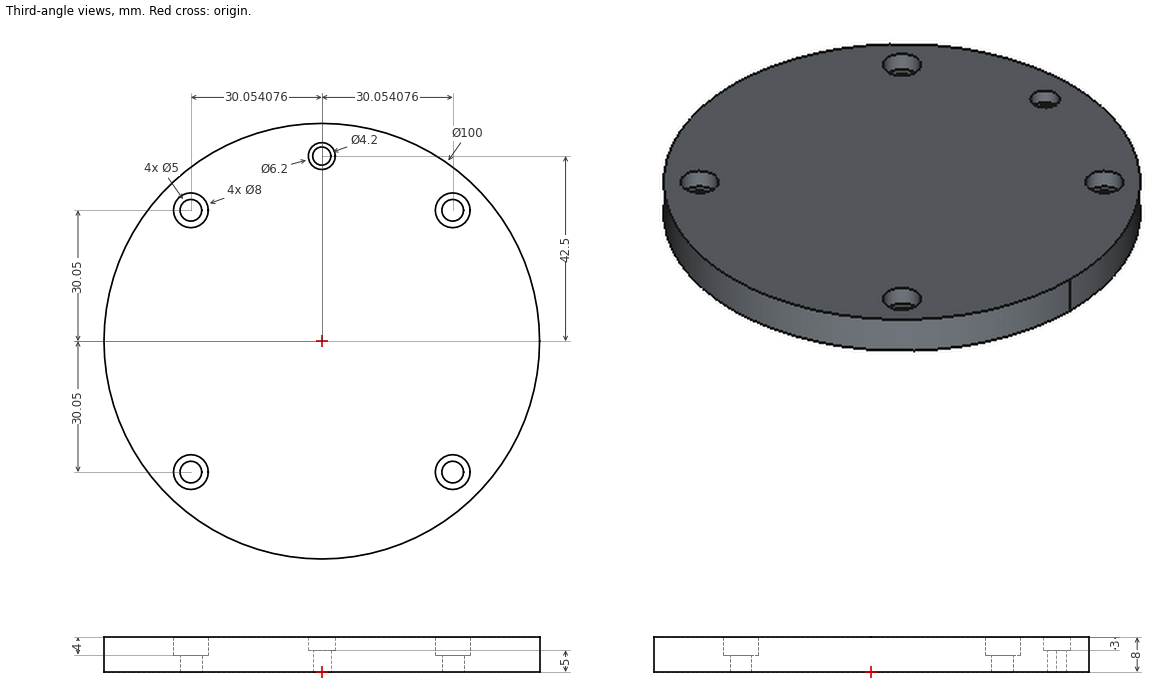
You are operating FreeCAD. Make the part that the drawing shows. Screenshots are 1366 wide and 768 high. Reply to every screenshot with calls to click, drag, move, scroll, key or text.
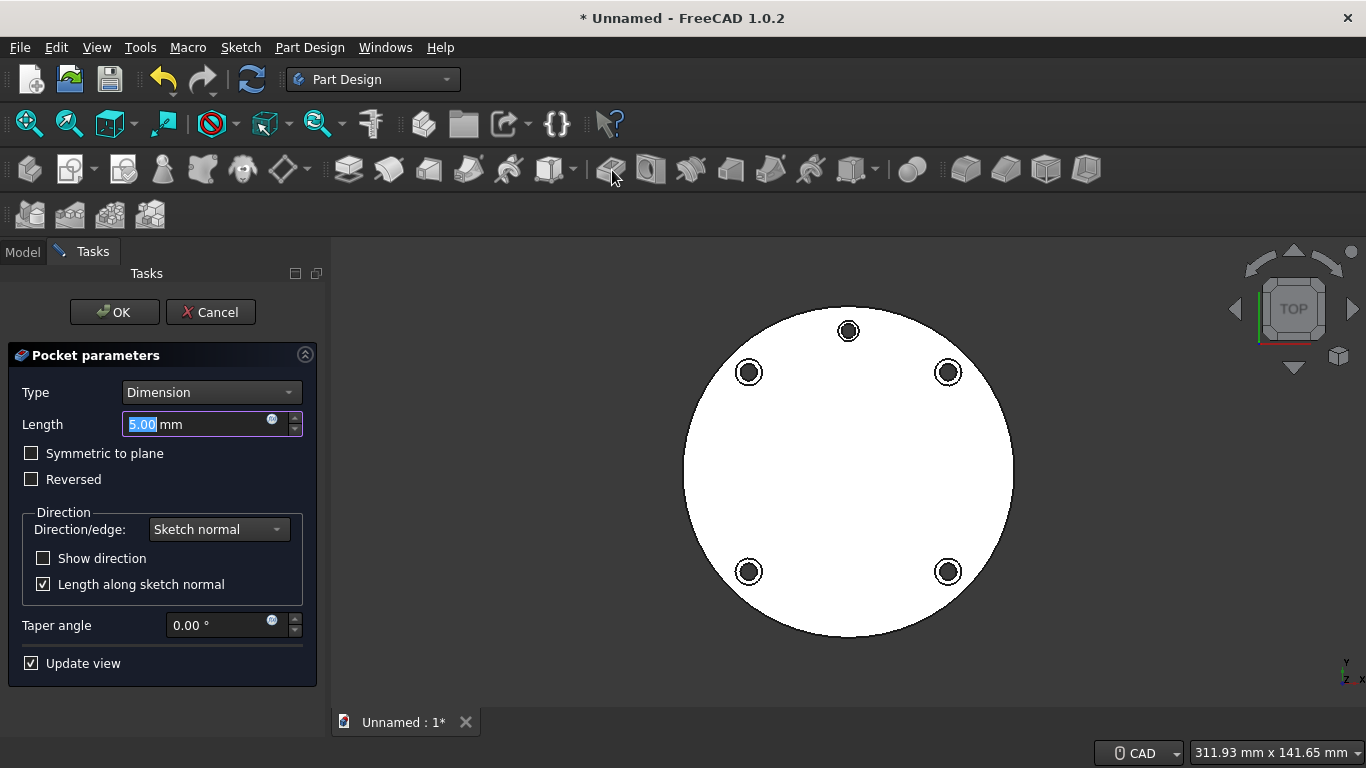
text(5)
key(Tab)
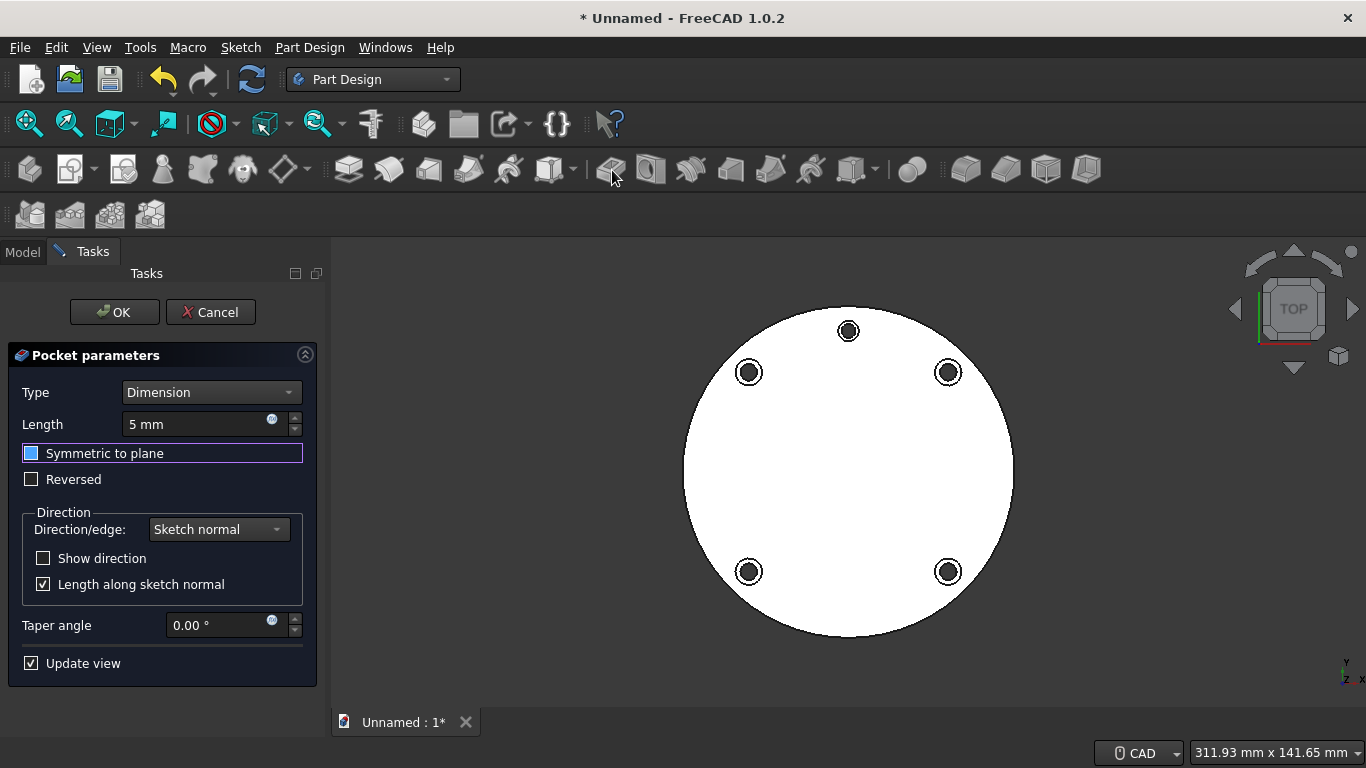
click(115, 312)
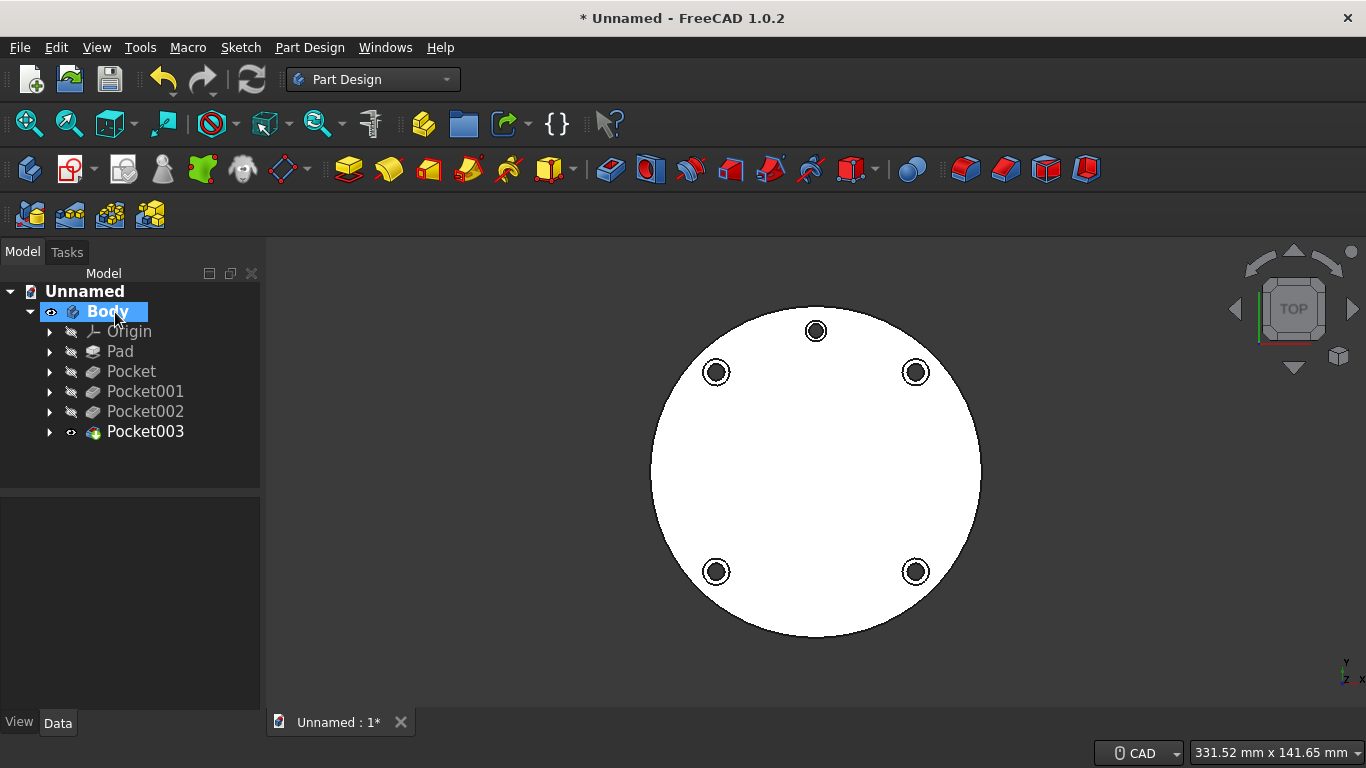
key(0)